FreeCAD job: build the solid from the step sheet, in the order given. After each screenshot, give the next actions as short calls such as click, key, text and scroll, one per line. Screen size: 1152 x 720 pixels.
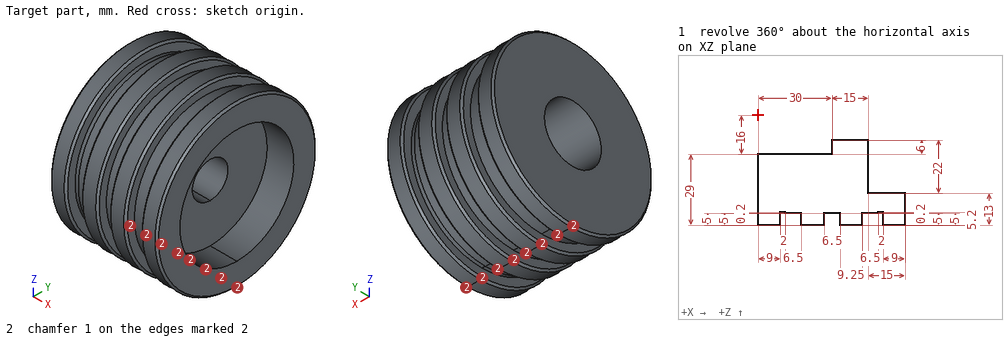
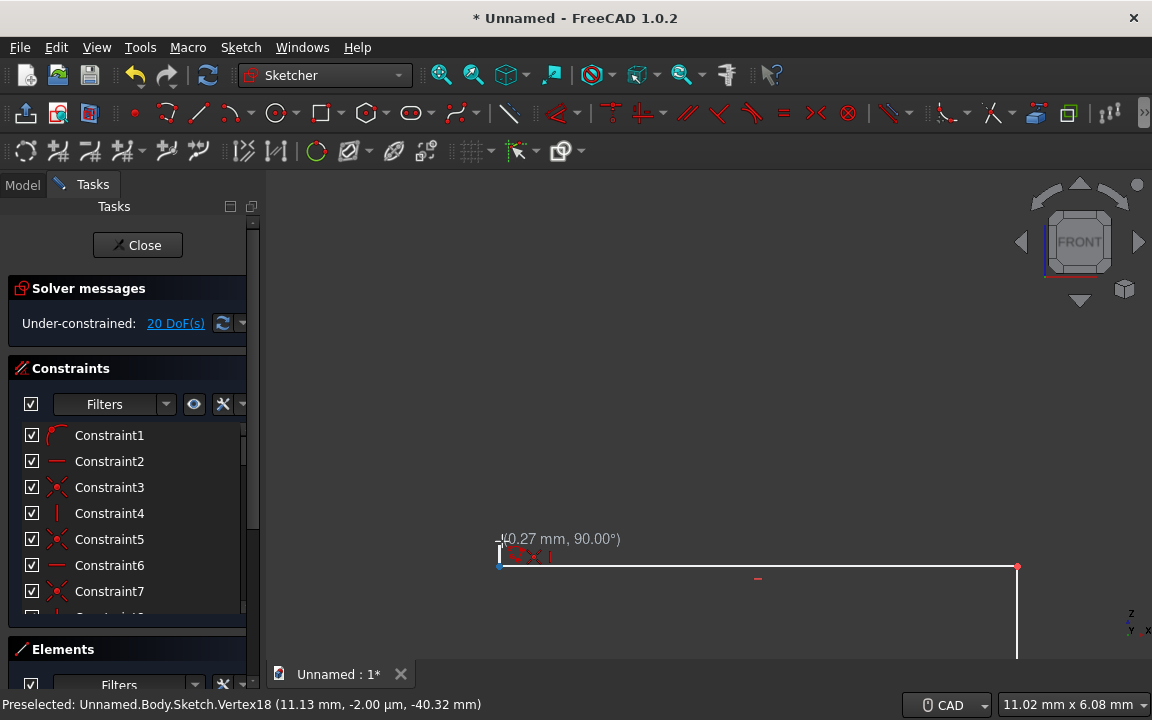
click(499, 535)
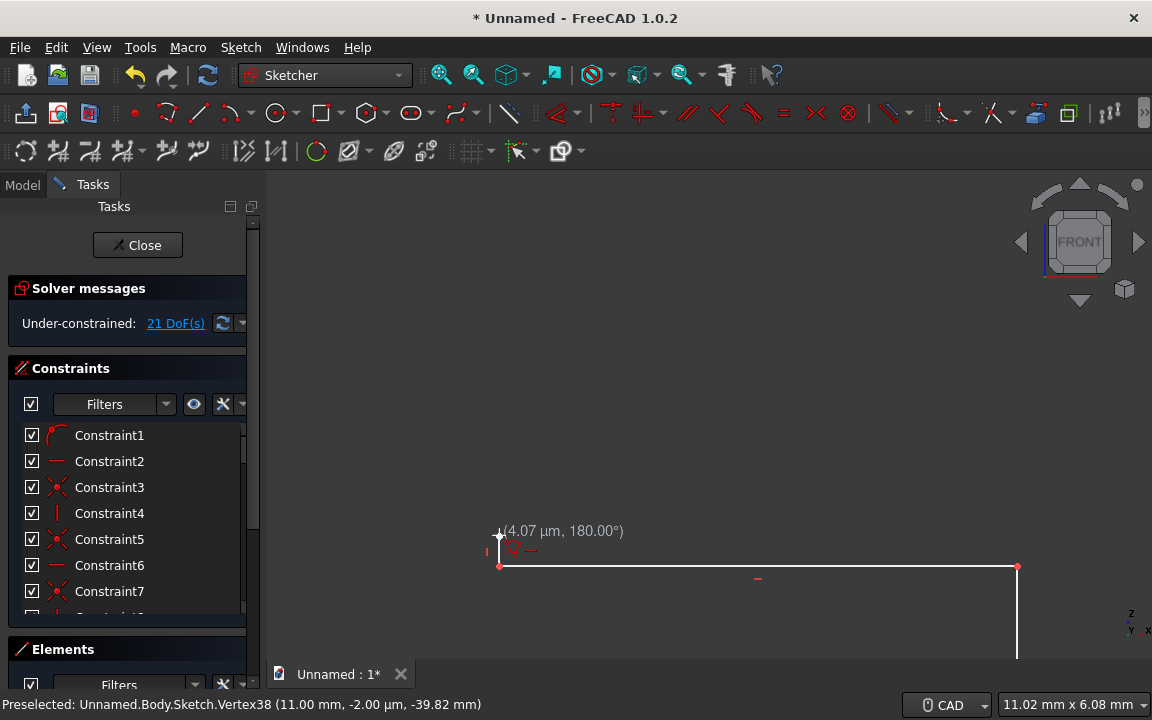
scroll(502, 541, down, 12)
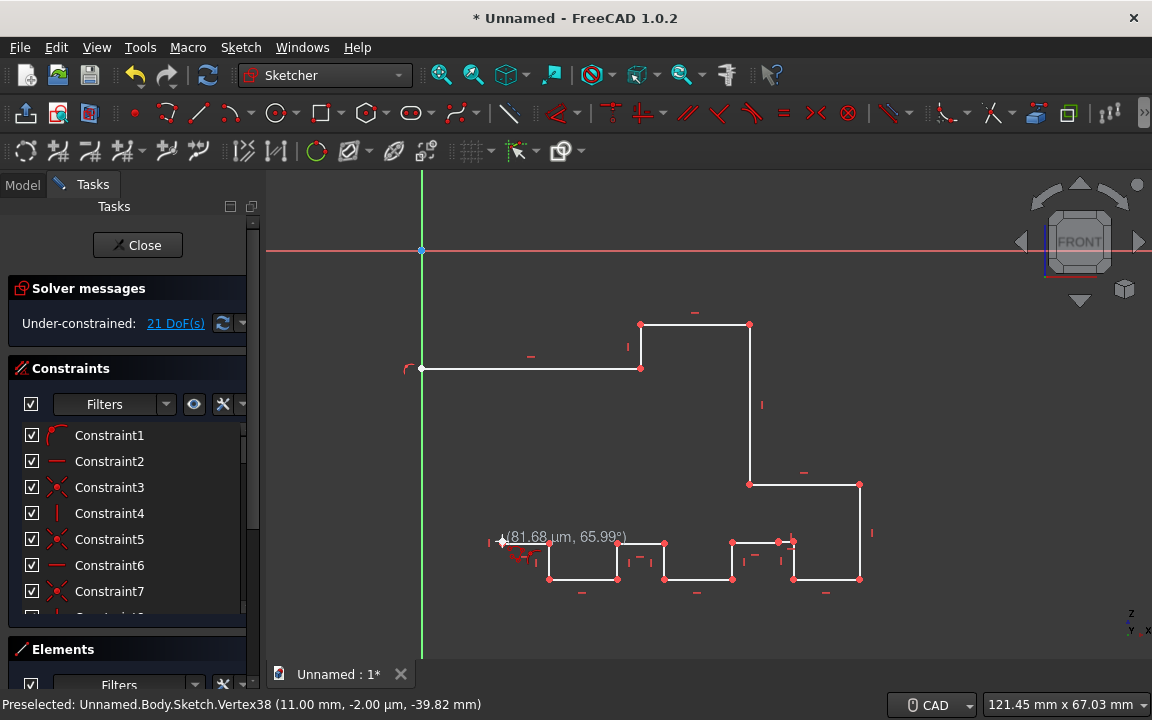
click(487, 541)
click(487, 579)
click(431, 579)
click(422, 369)
key(Escape)
key(Escape)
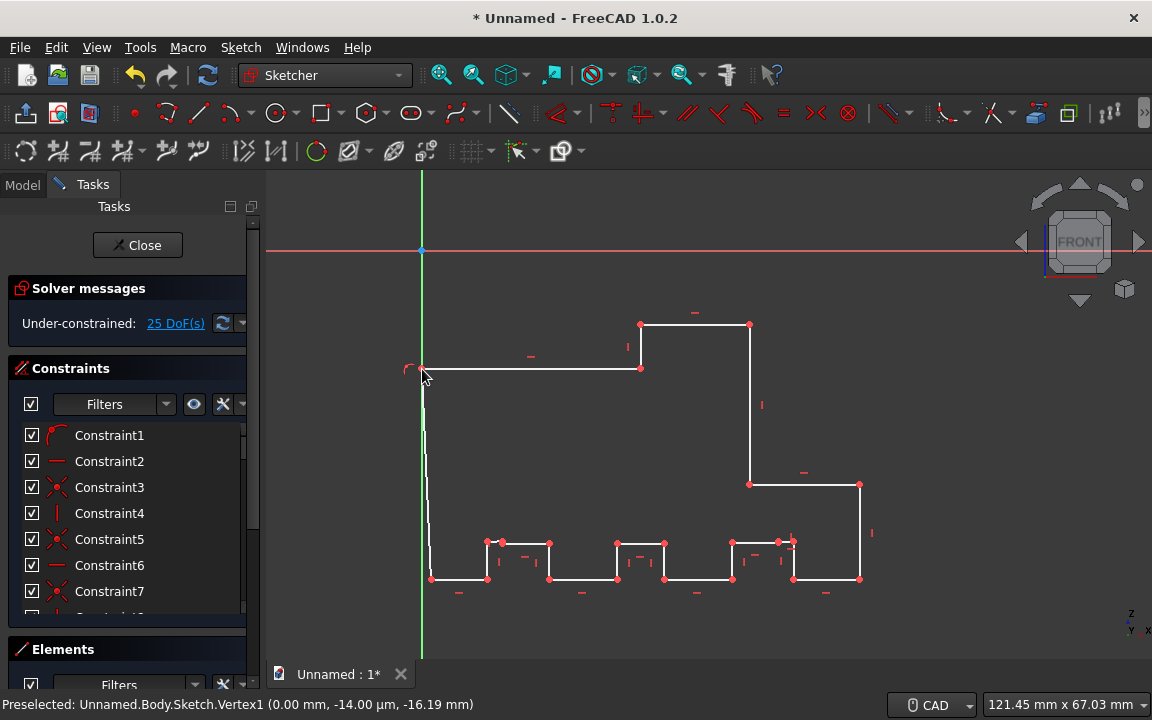
scroll(495, 542, up, 4)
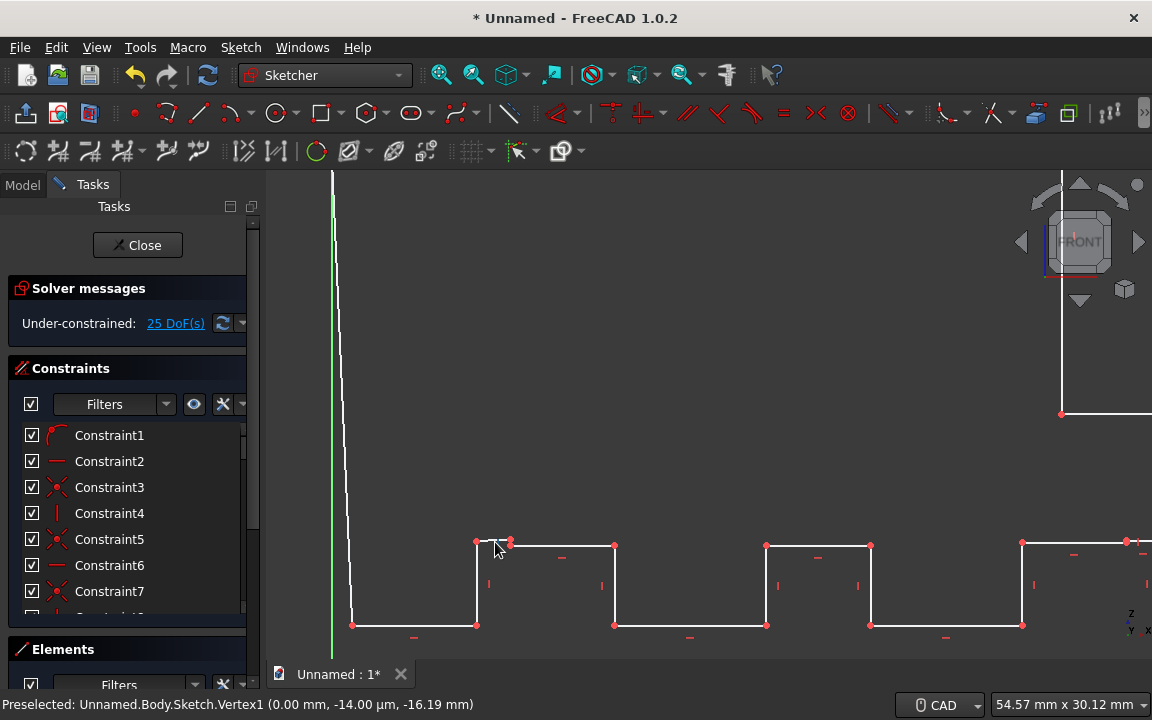
click(490, 540)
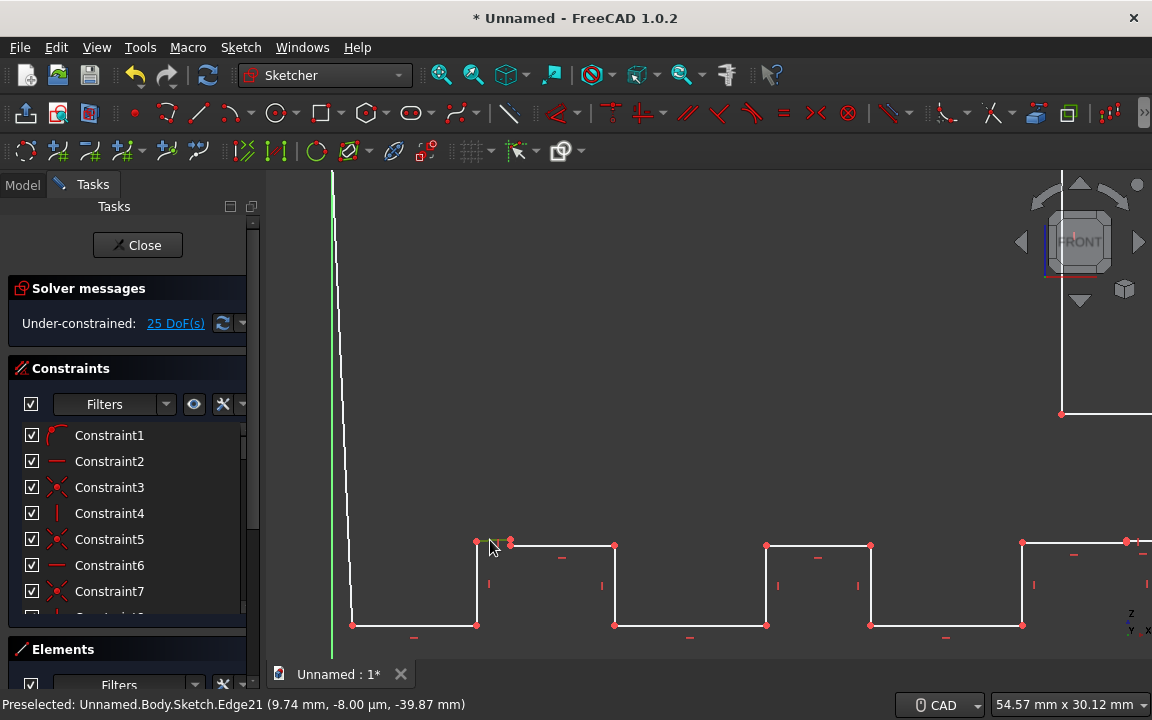
key(h)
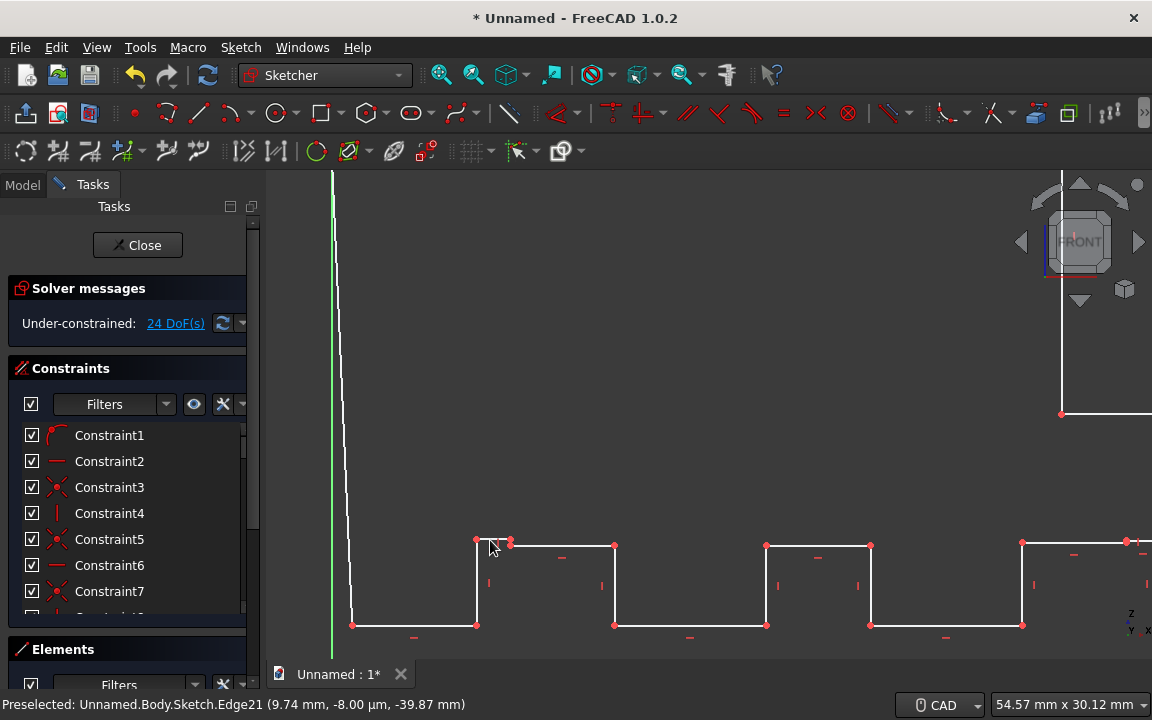
click(346, 485)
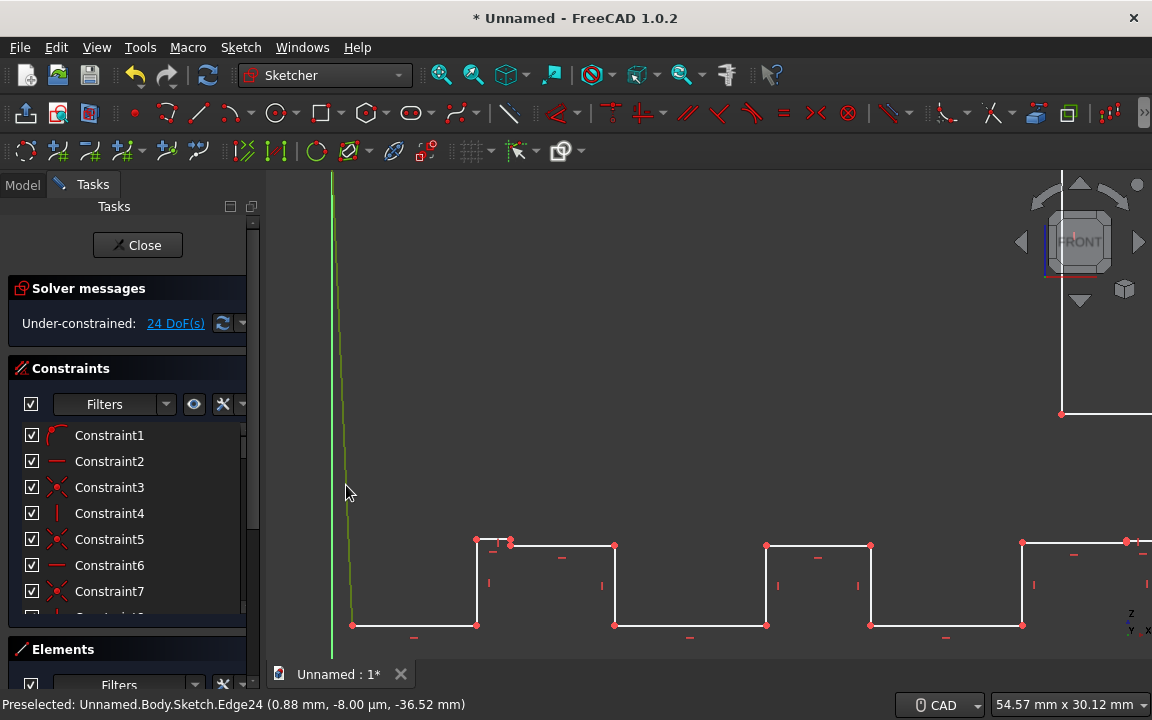
key(v)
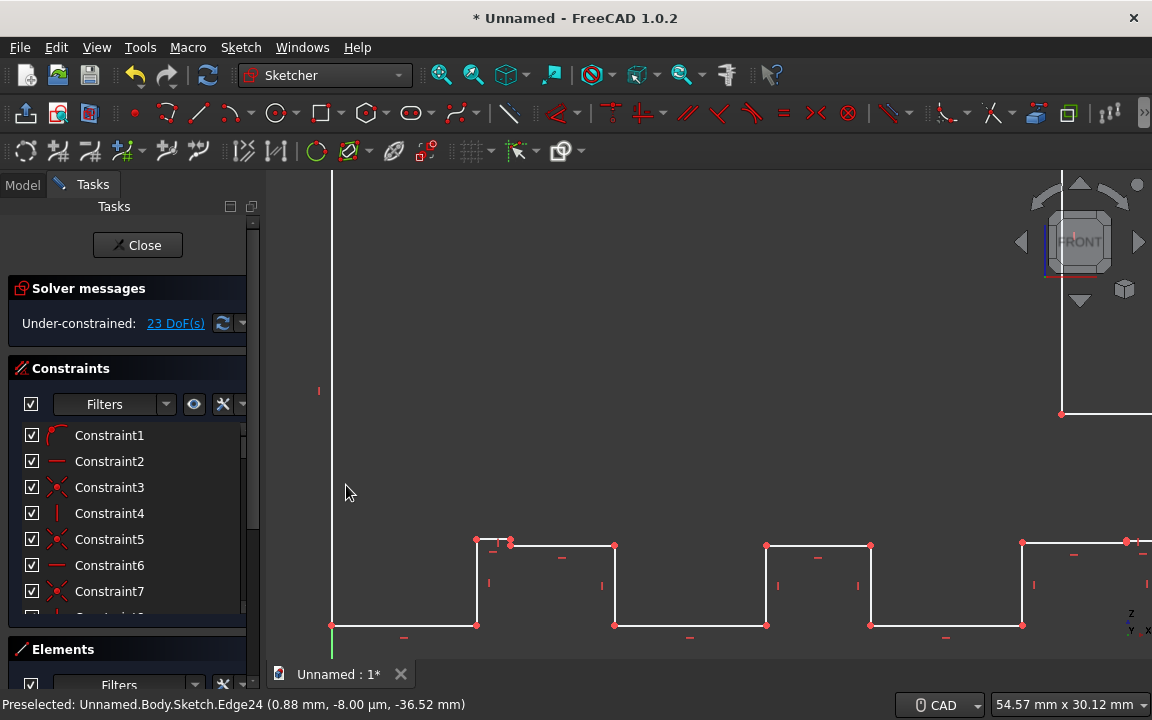
click(556, 114)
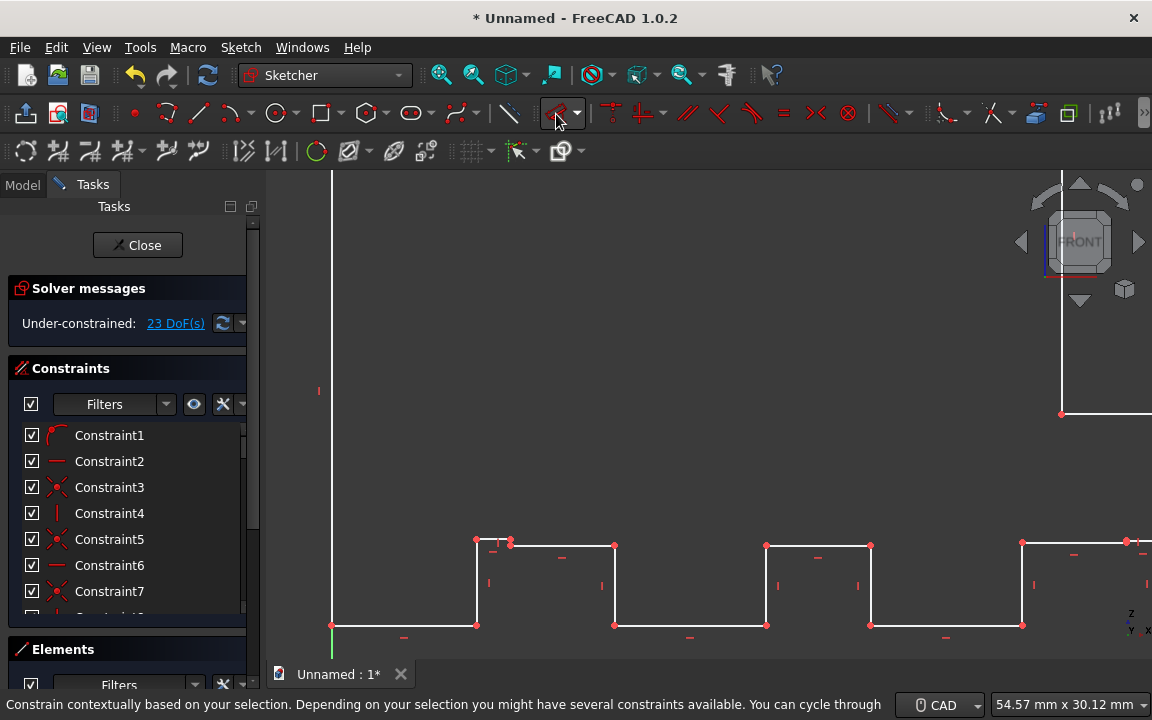
scroll(495, 542, down, 4)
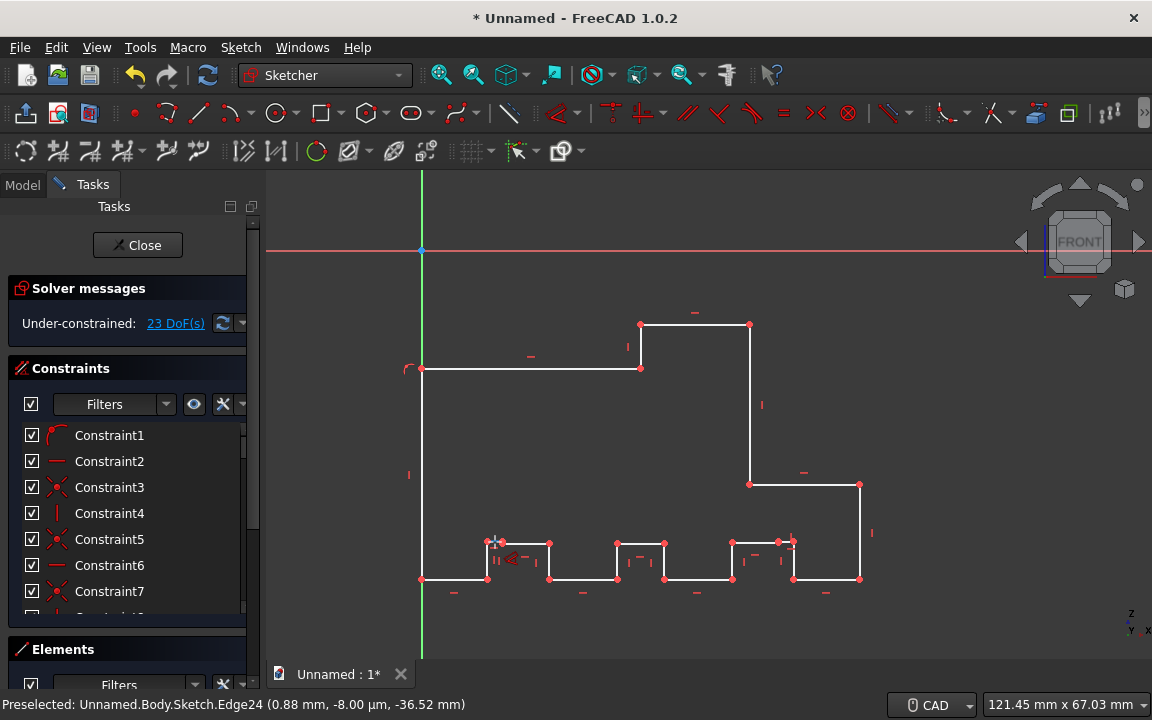
click(641, 356)
click(675, 347)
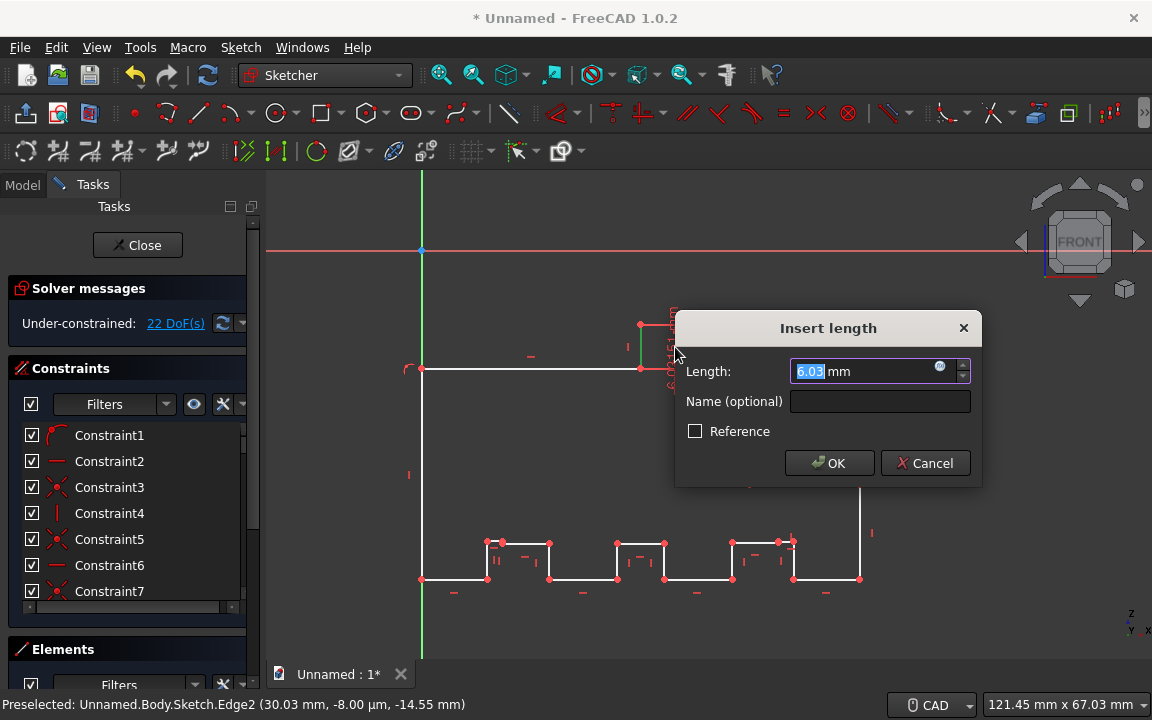
text(6)
key(Return)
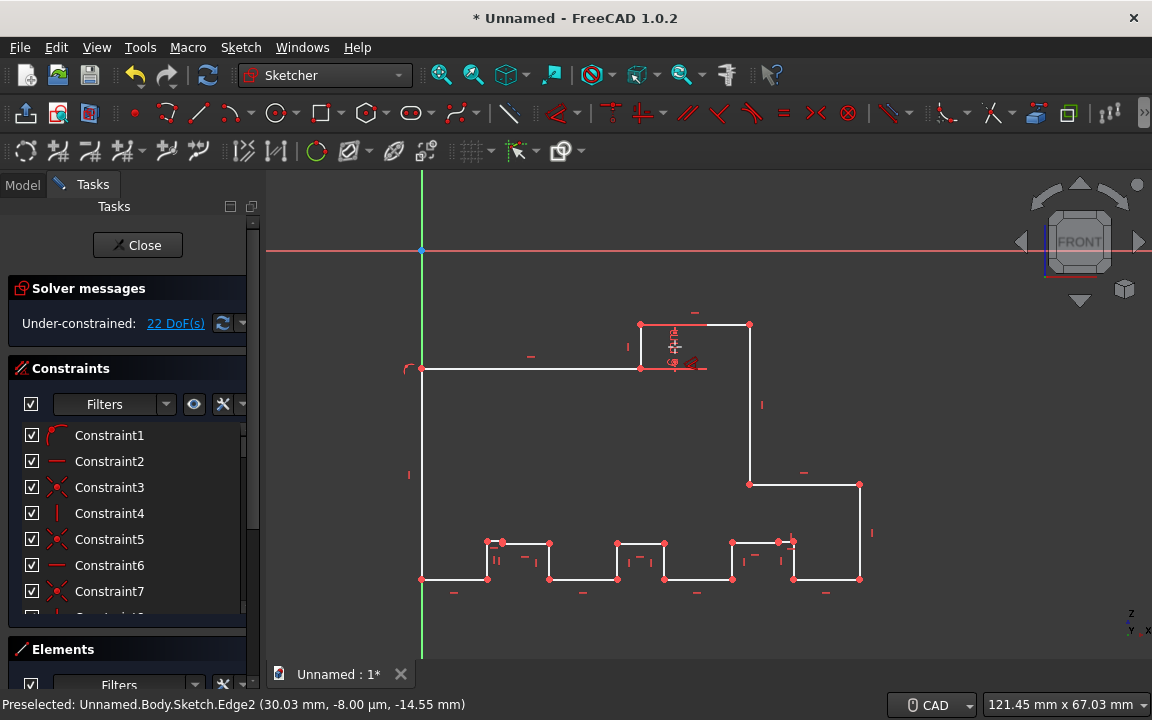
click(840, 580)
click(827, 614)